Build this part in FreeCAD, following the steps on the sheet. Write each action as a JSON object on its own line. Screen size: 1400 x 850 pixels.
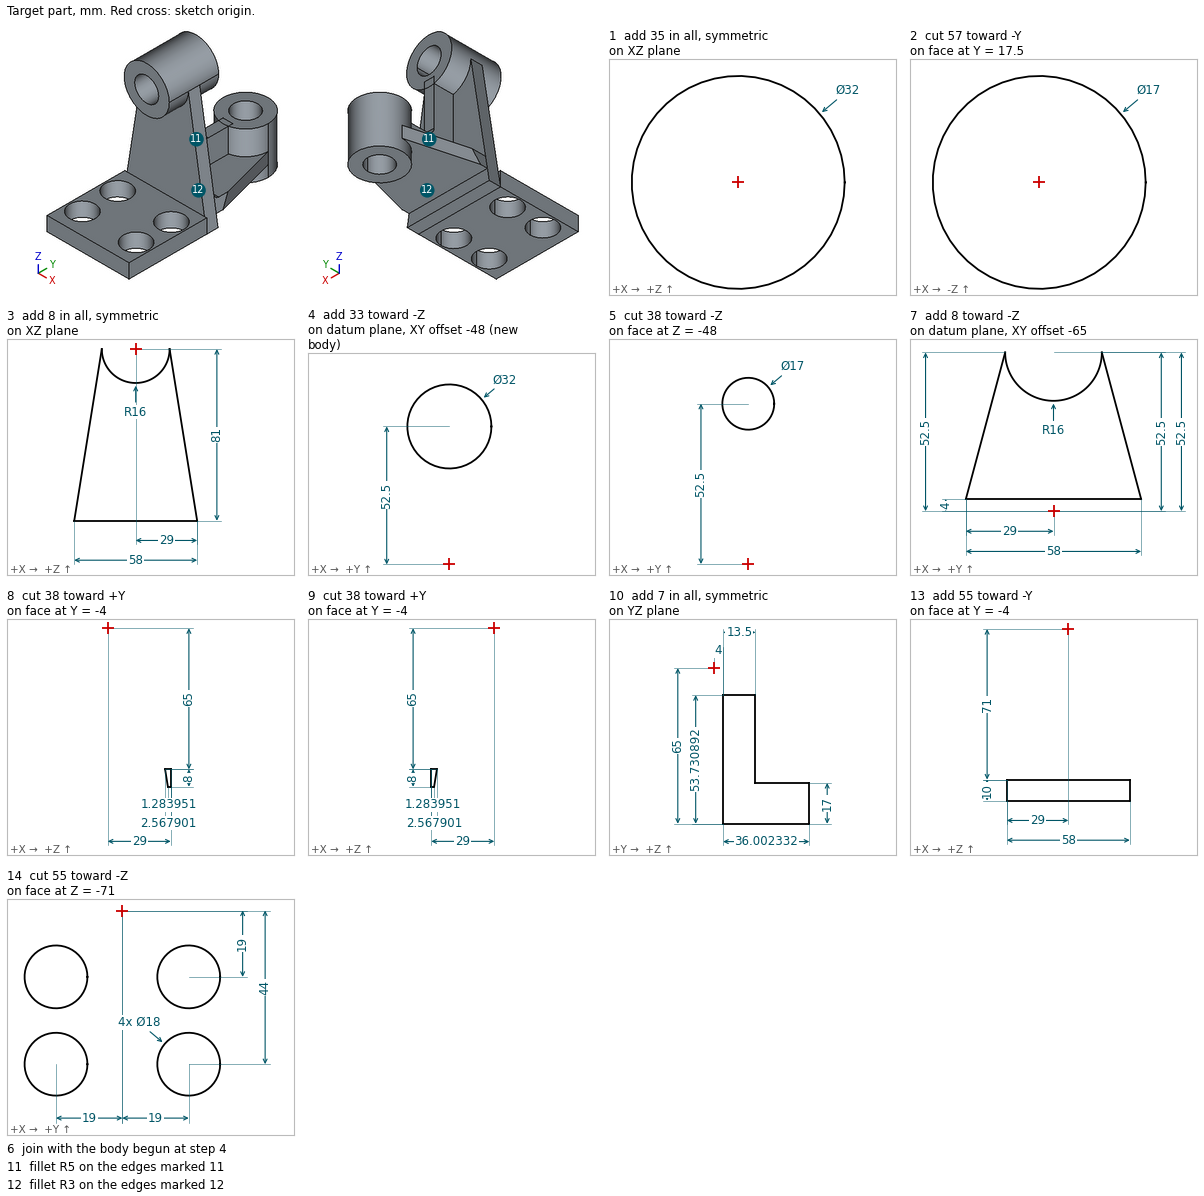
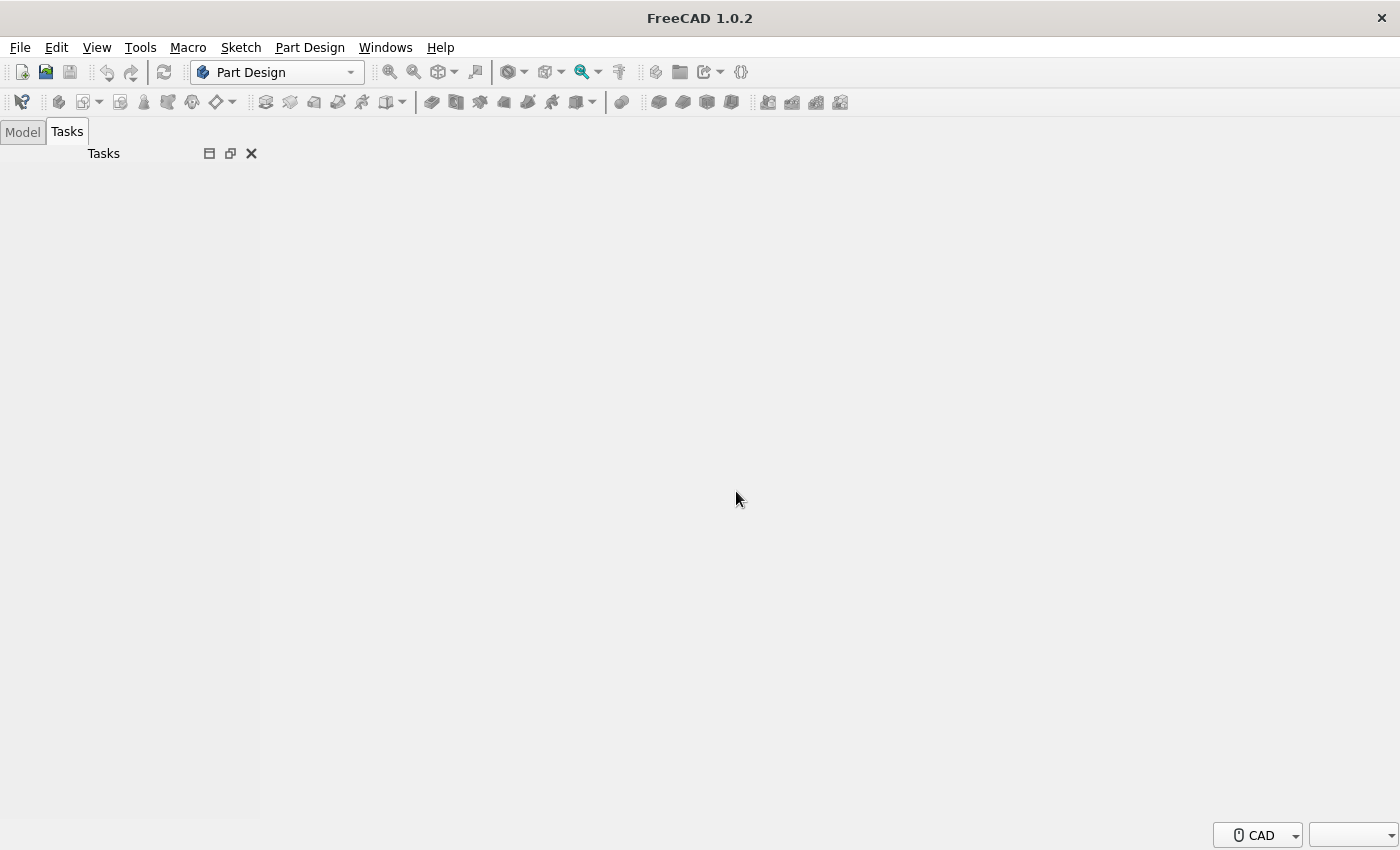
{"action": "key", "text": "ctrl+n"}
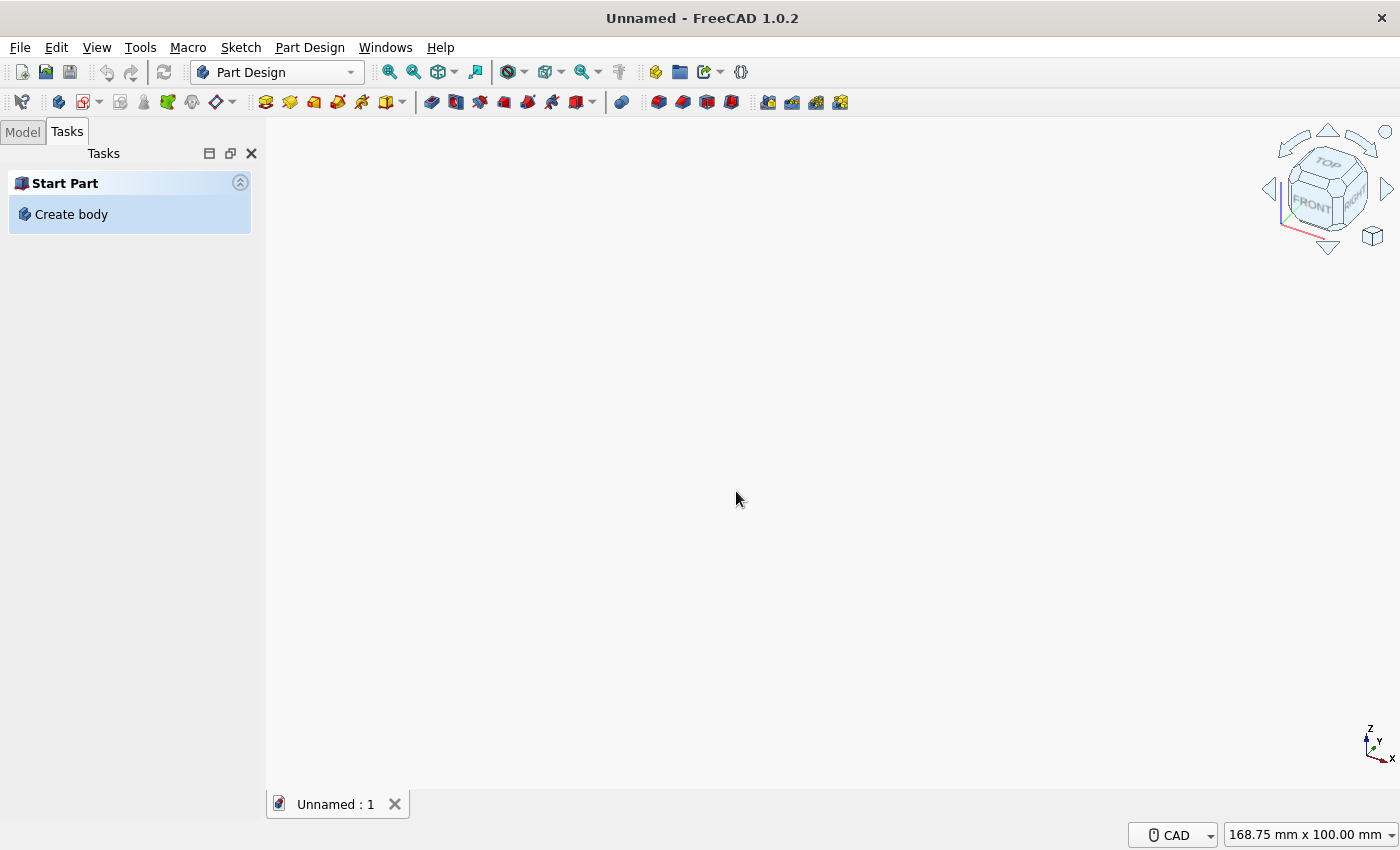
{"action": "left_click", "coordinate": [84, 102]}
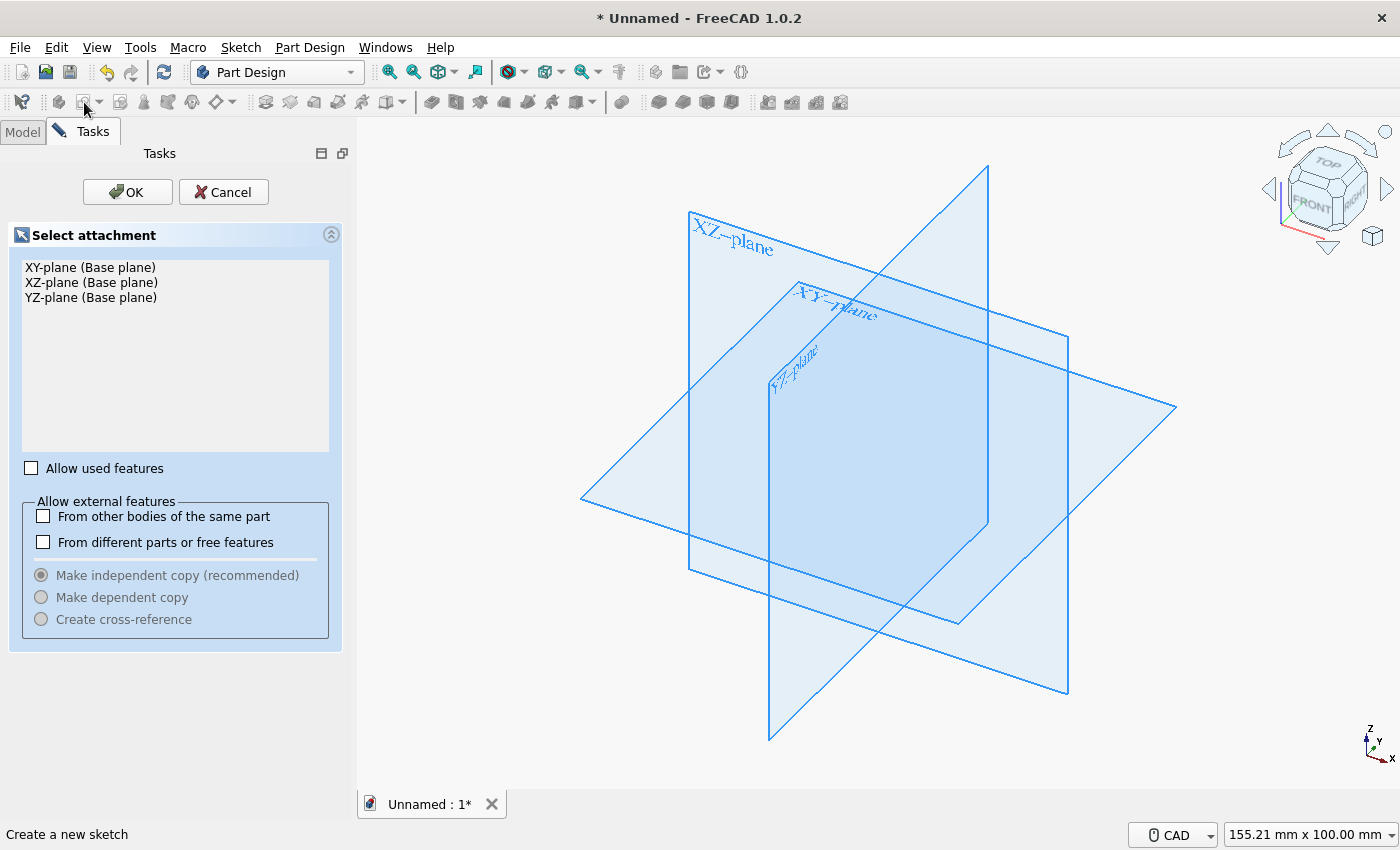
{"action": "left_click", "coordinate": [82, 282]}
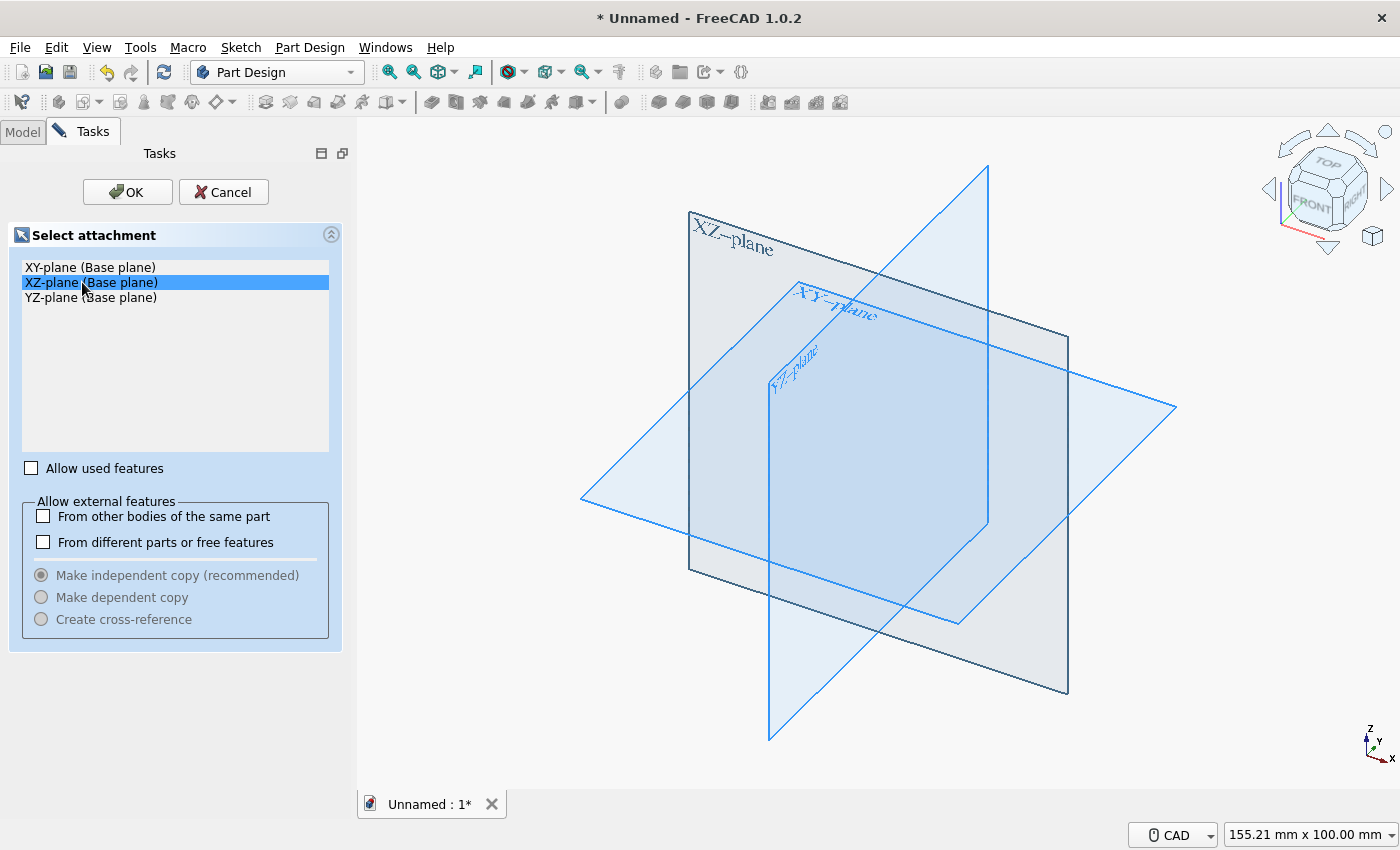
{"action": "left_click", "coordinate": [128, 192]}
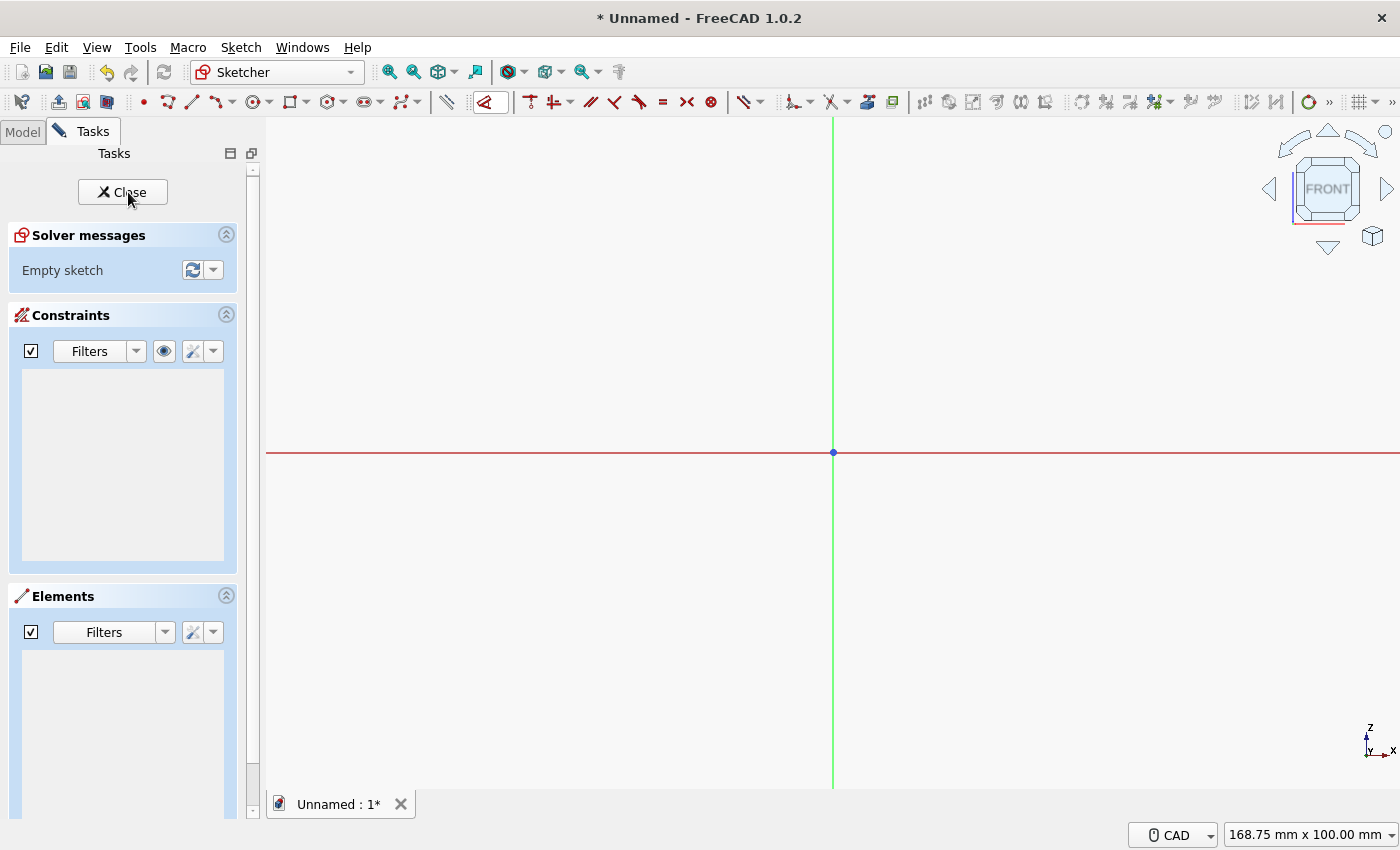
{"action": "scroll", "coordinate": [889, 453], "scroll_direction": "up", "scroll_amount": 4}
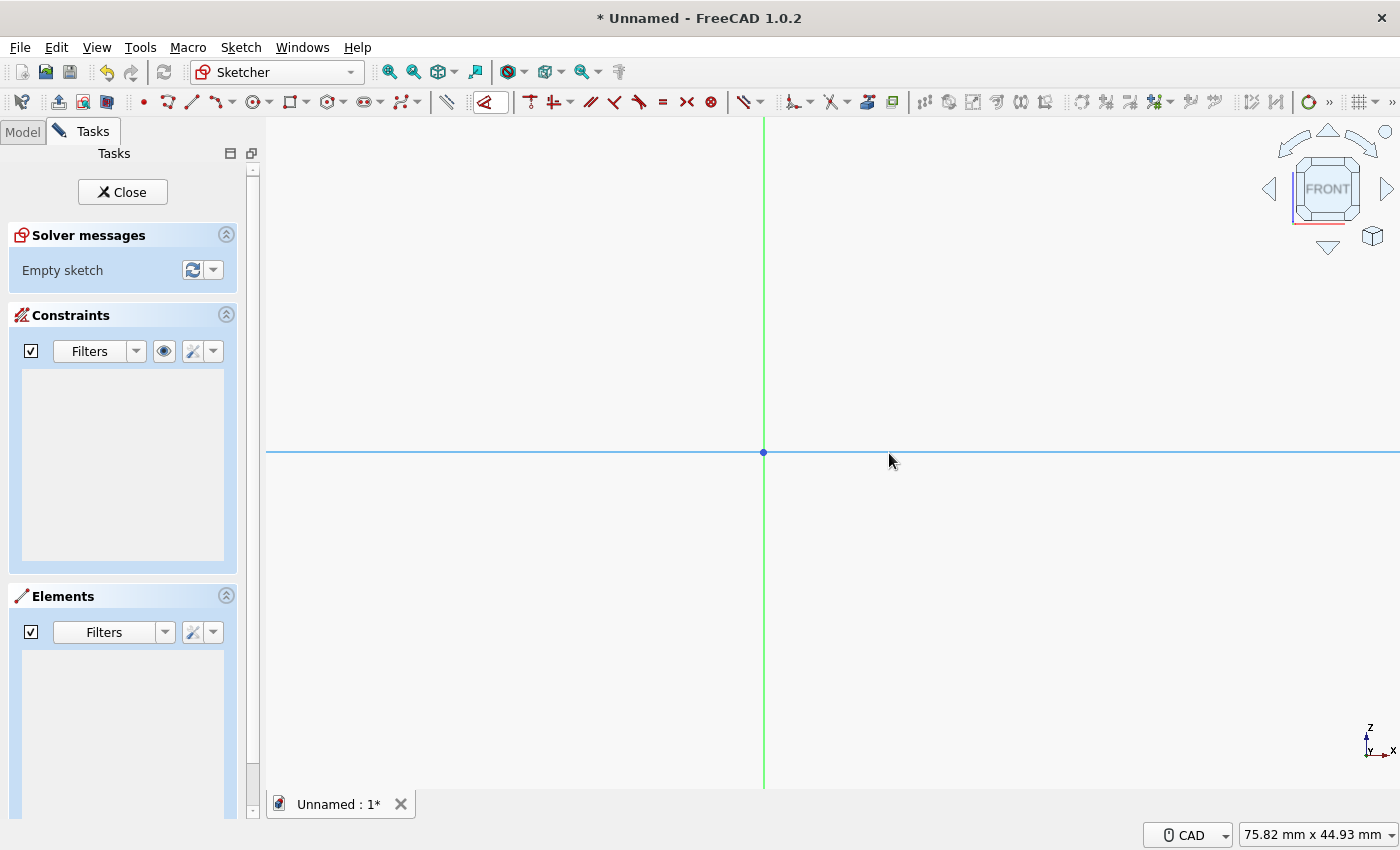
{"action": "key", "text": "g c"}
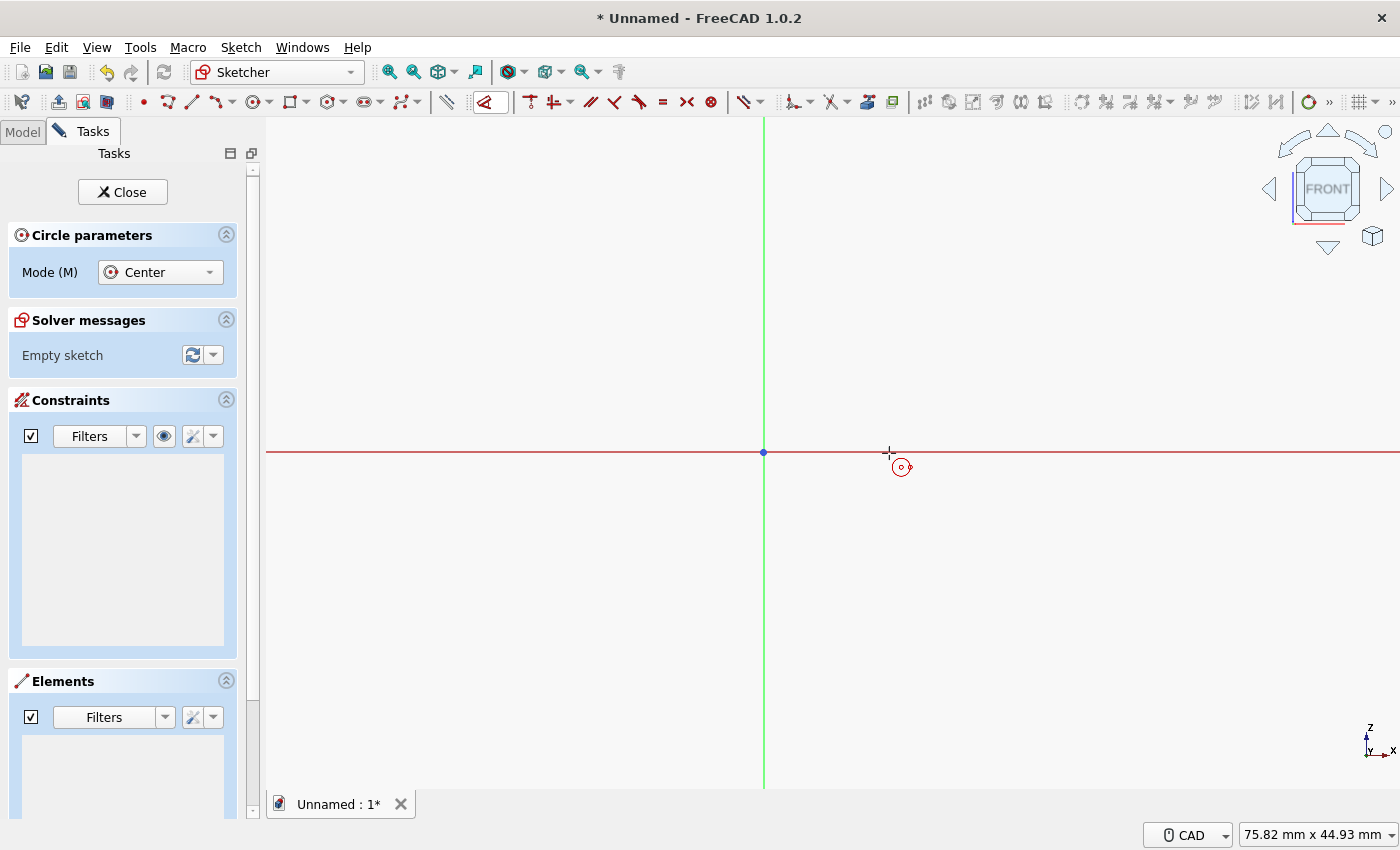
{"action": "left_click", "coordinate": [764, 452]}
{"action": "left_click", "coordinate": [933, 283]}
{"action": "key", "text": "Escape"}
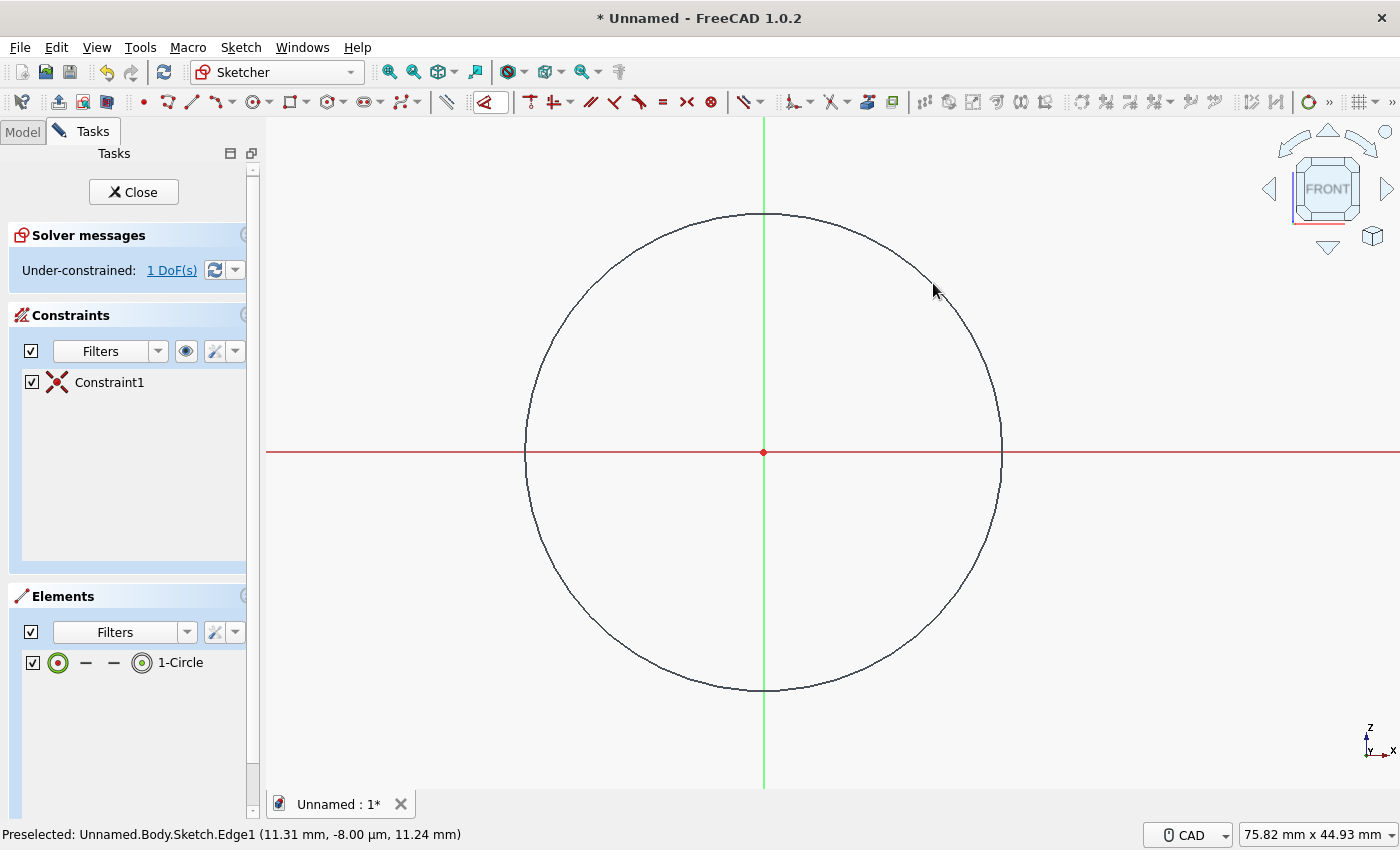
{"action": "key", "text": "d"}